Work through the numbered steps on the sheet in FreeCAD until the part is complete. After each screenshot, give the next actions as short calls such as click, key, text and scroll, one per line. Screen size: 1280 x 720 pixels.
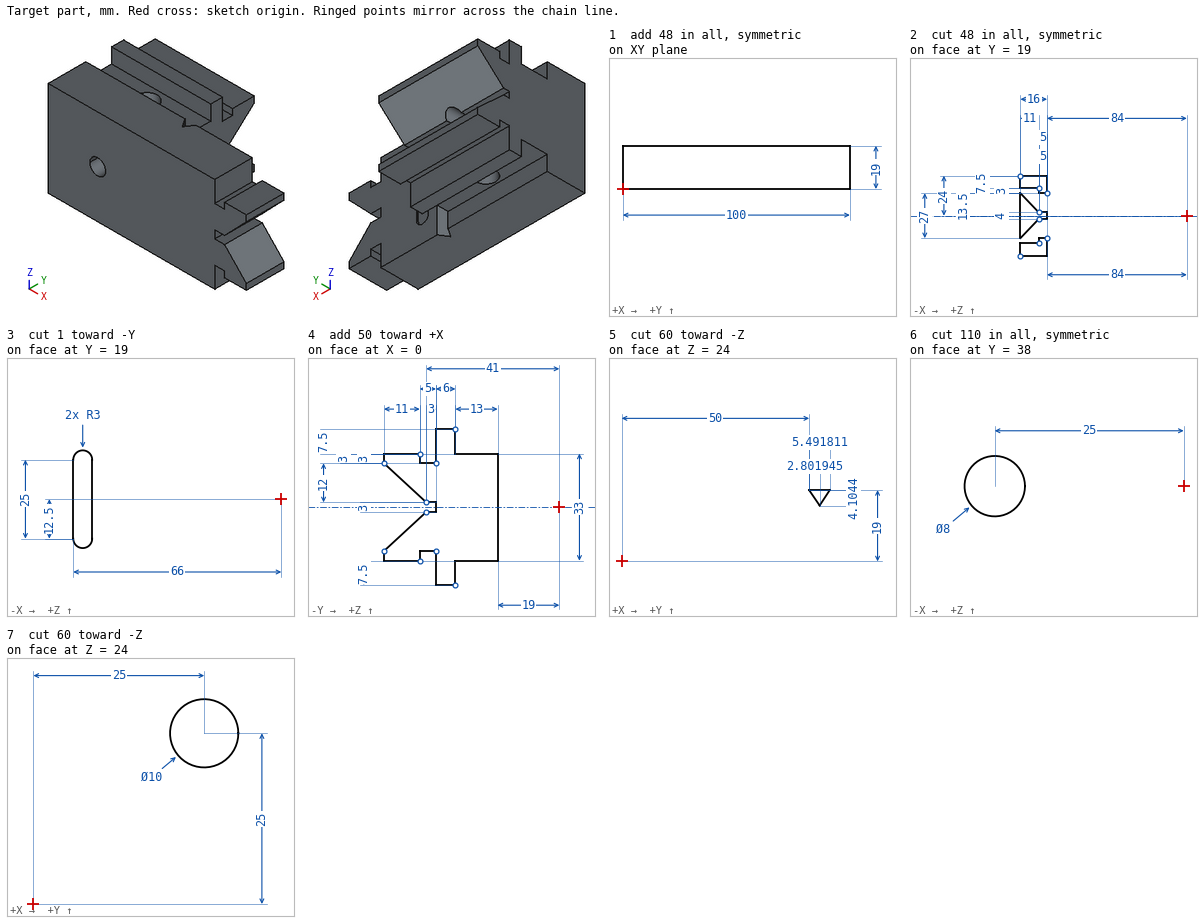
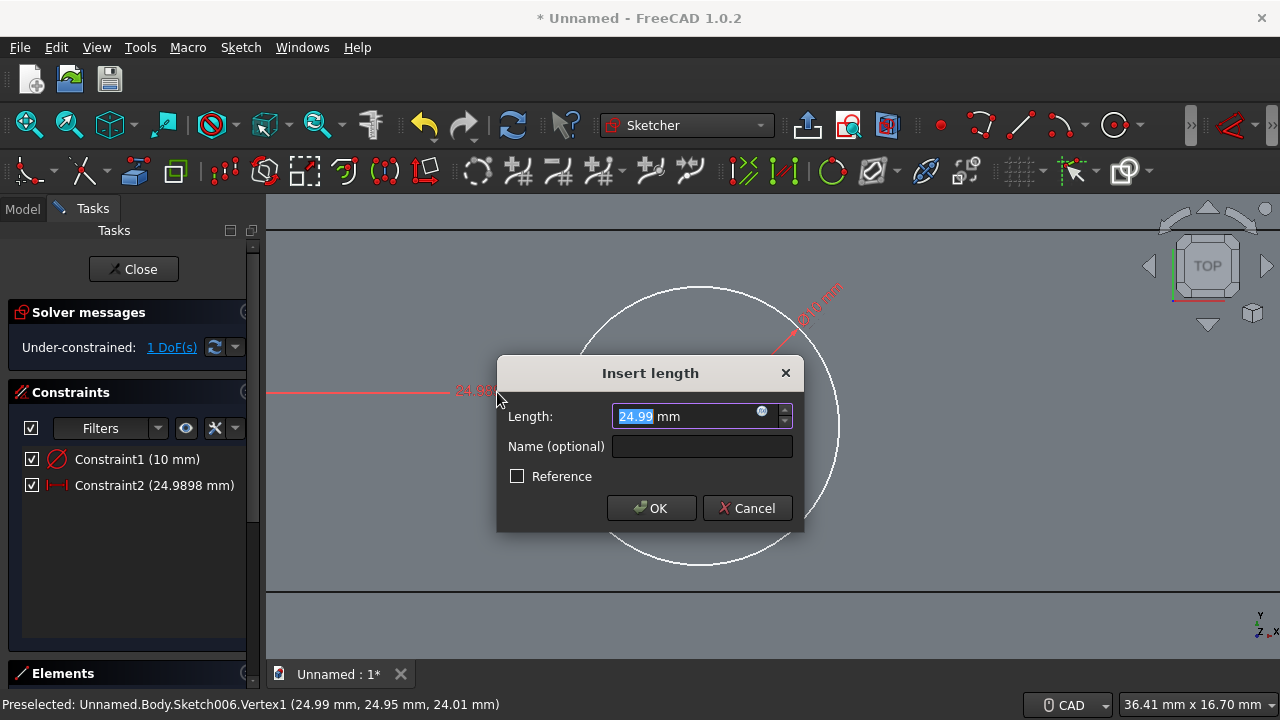
text(25)
key(Return)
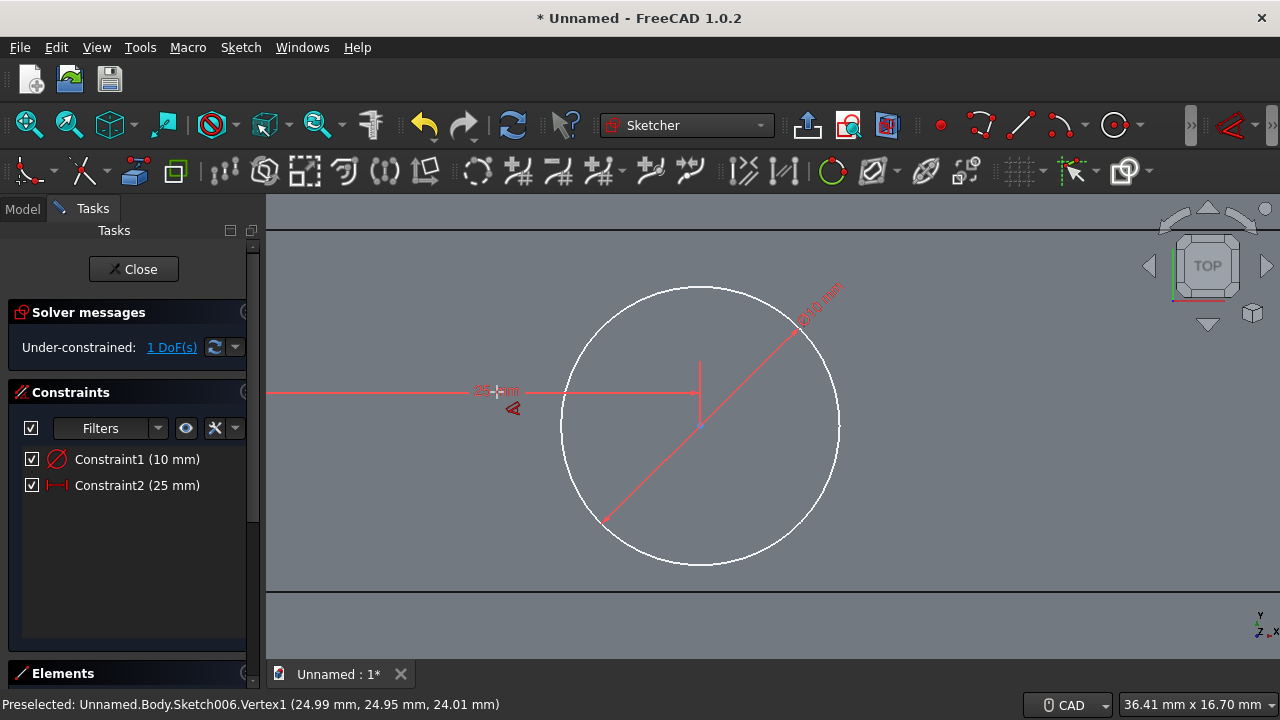
click(700, 426)
click(734, 528)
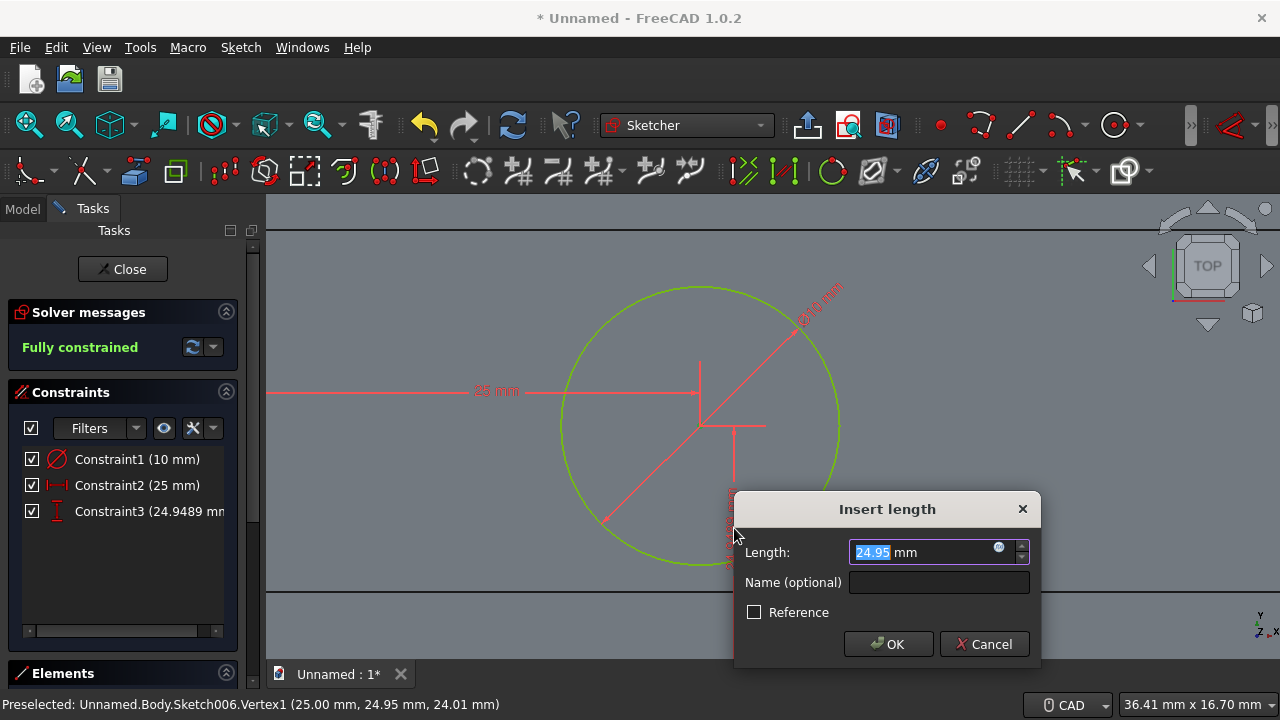
text(25)
key(Return)
key(Escape)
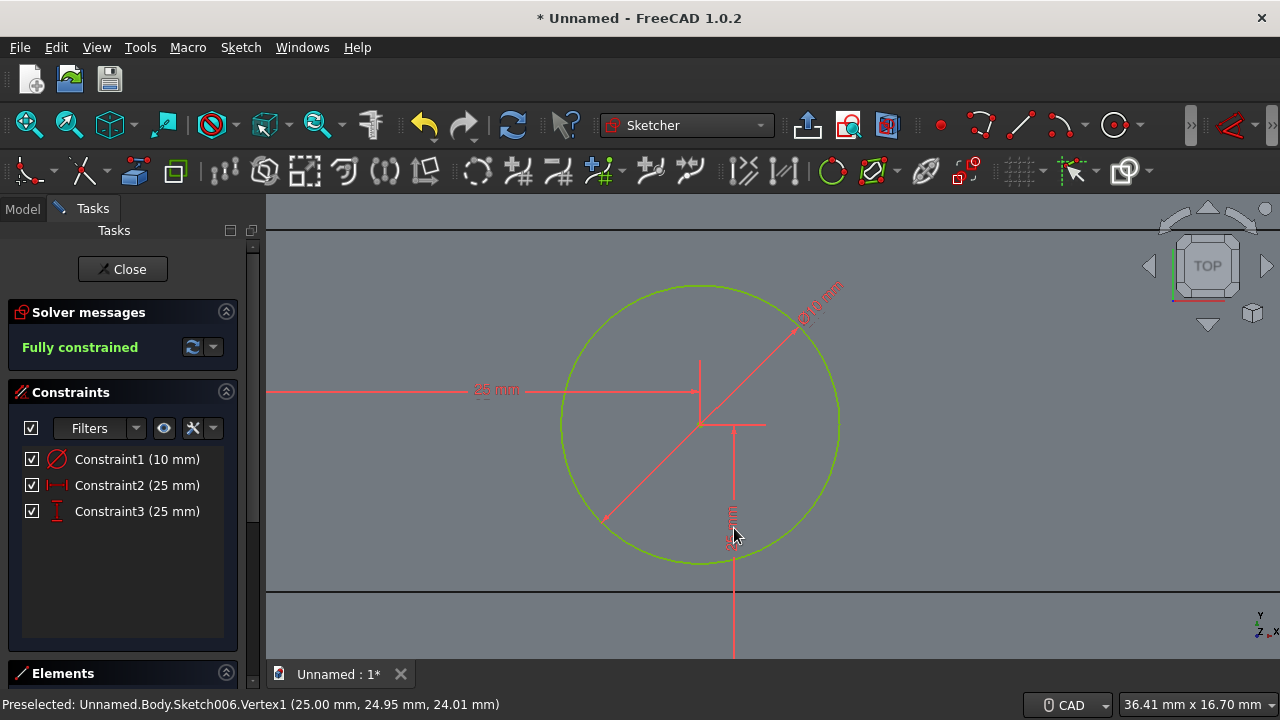
click(123, 269)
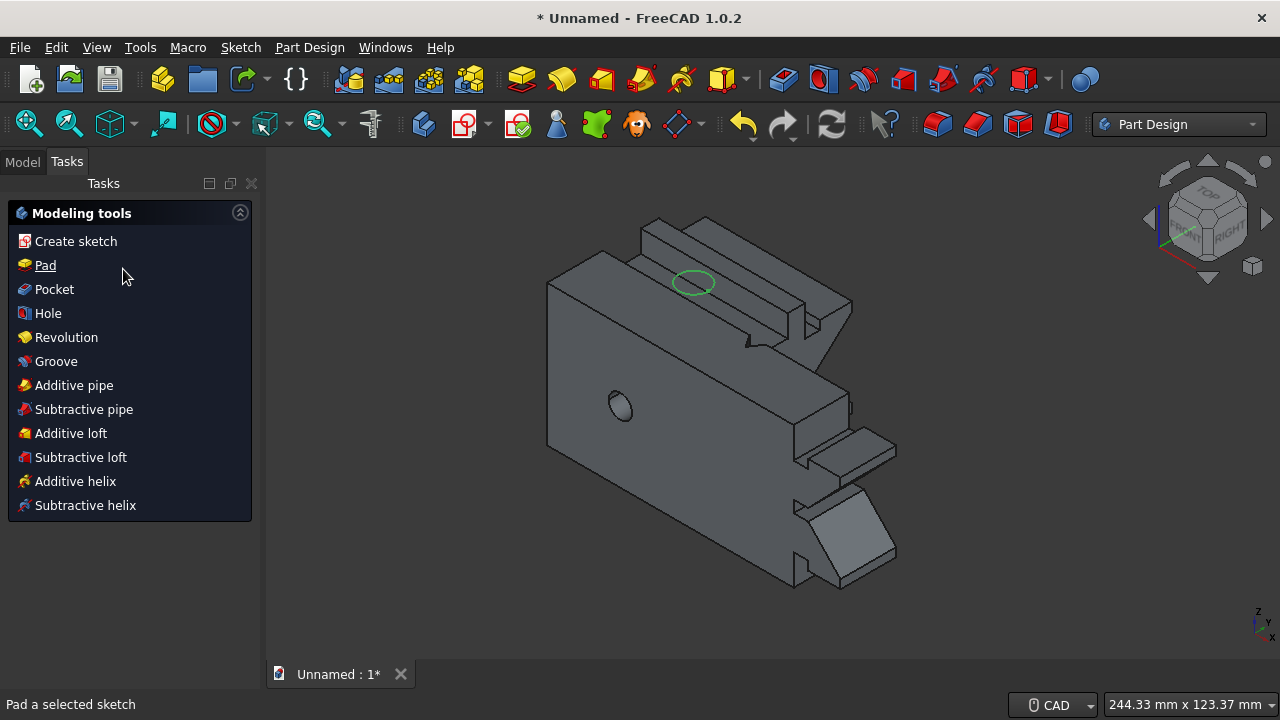
click(784, 80)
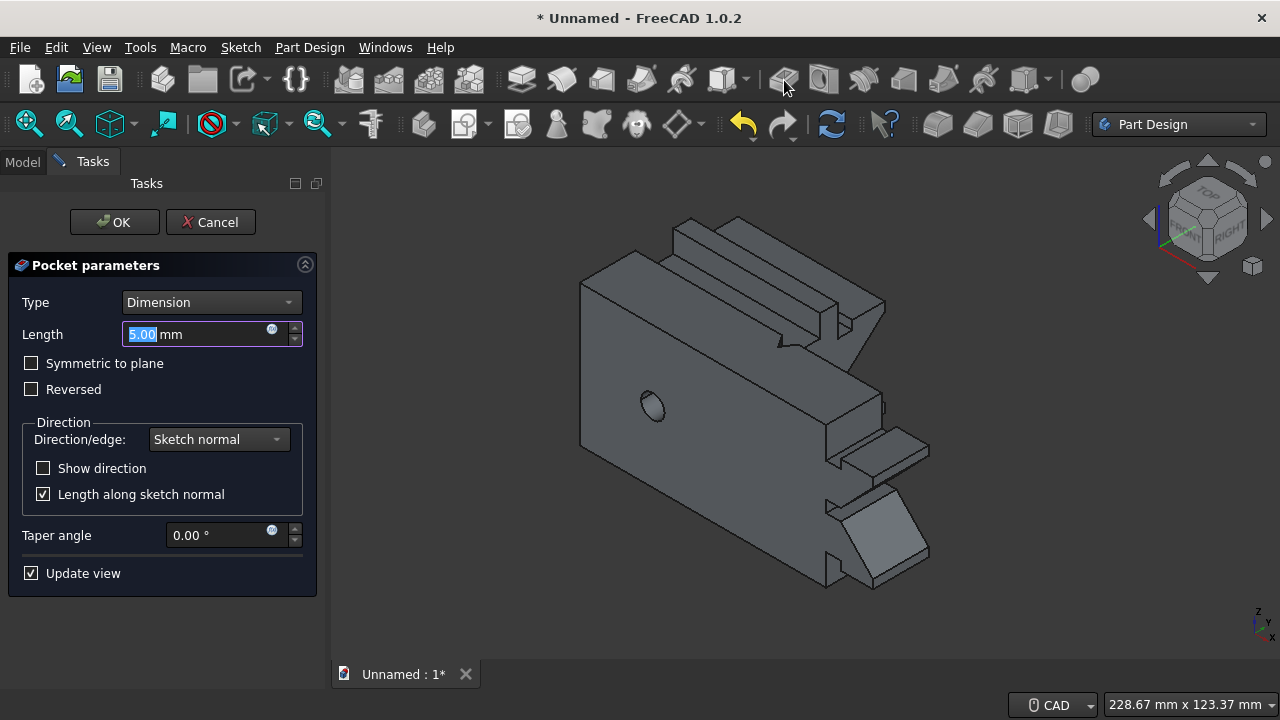
text(60)
key(Tab)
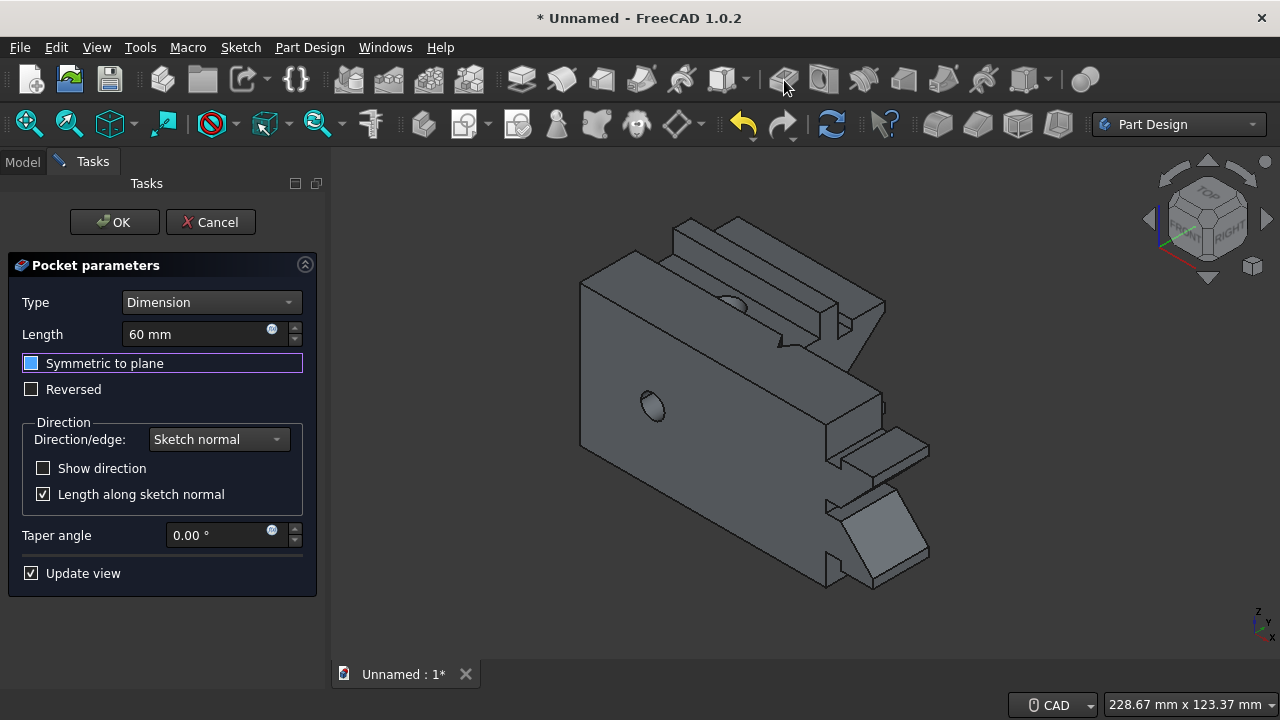
click(115, 222)